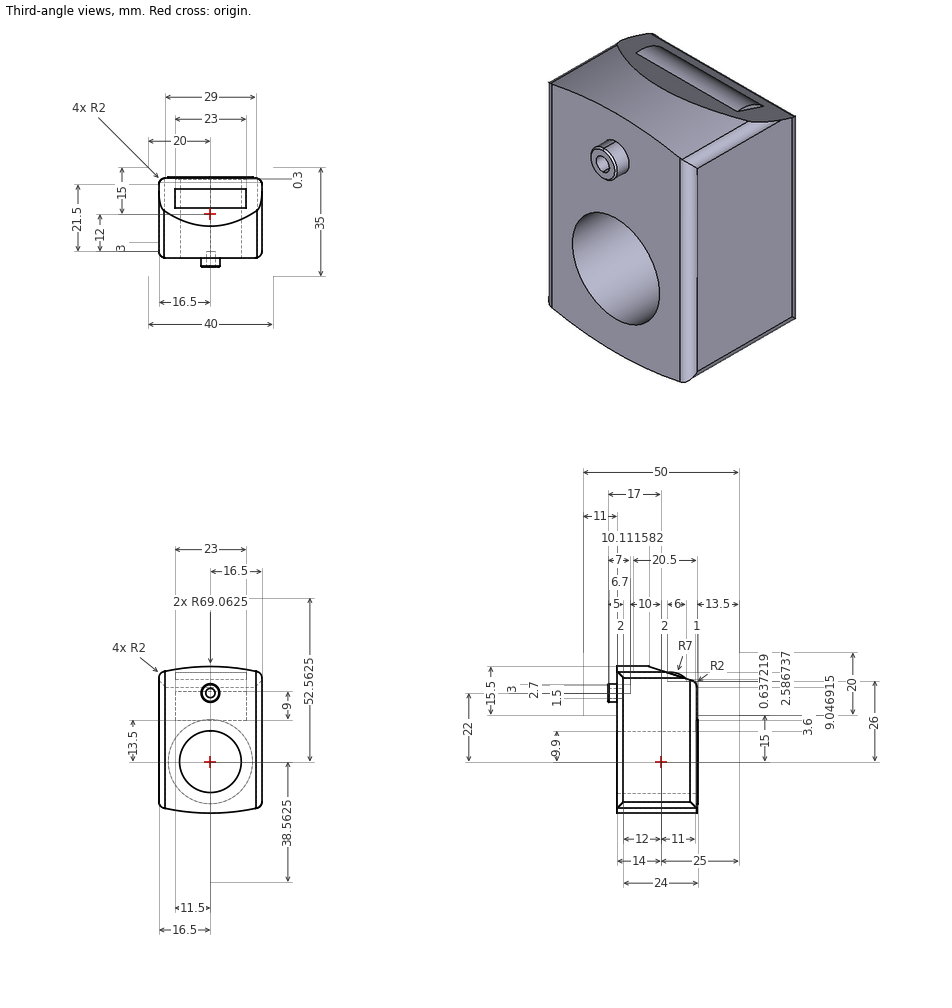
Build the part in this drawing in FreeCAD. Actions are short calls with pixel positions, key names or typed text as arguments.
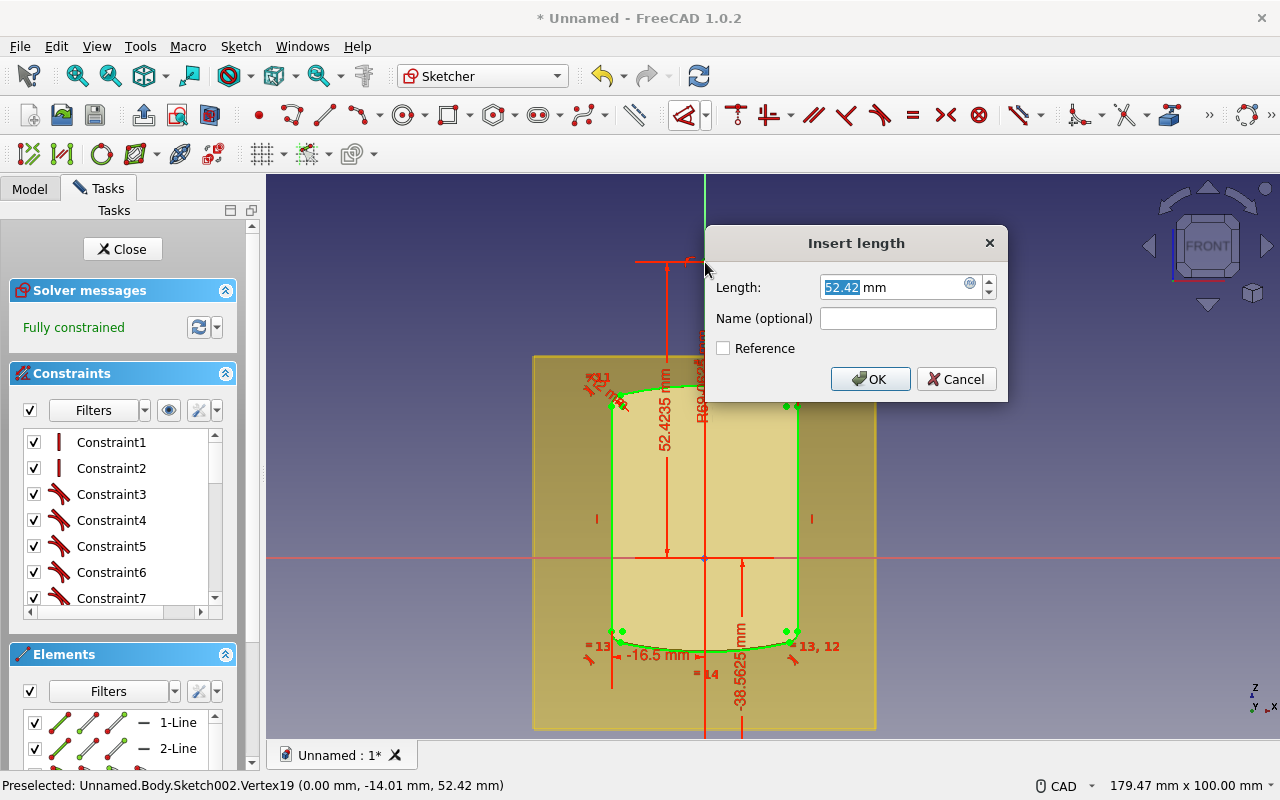
text(52.5625)
key(Return)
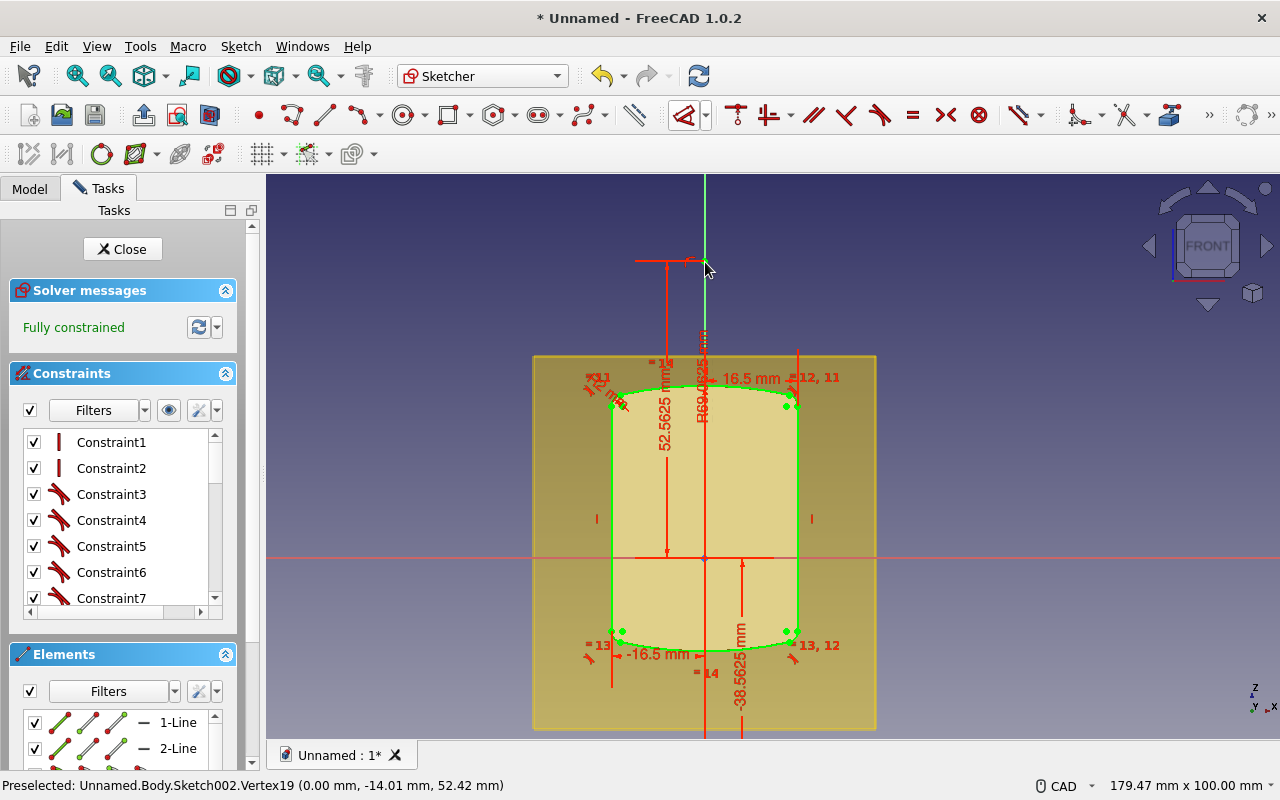
click(123, 249)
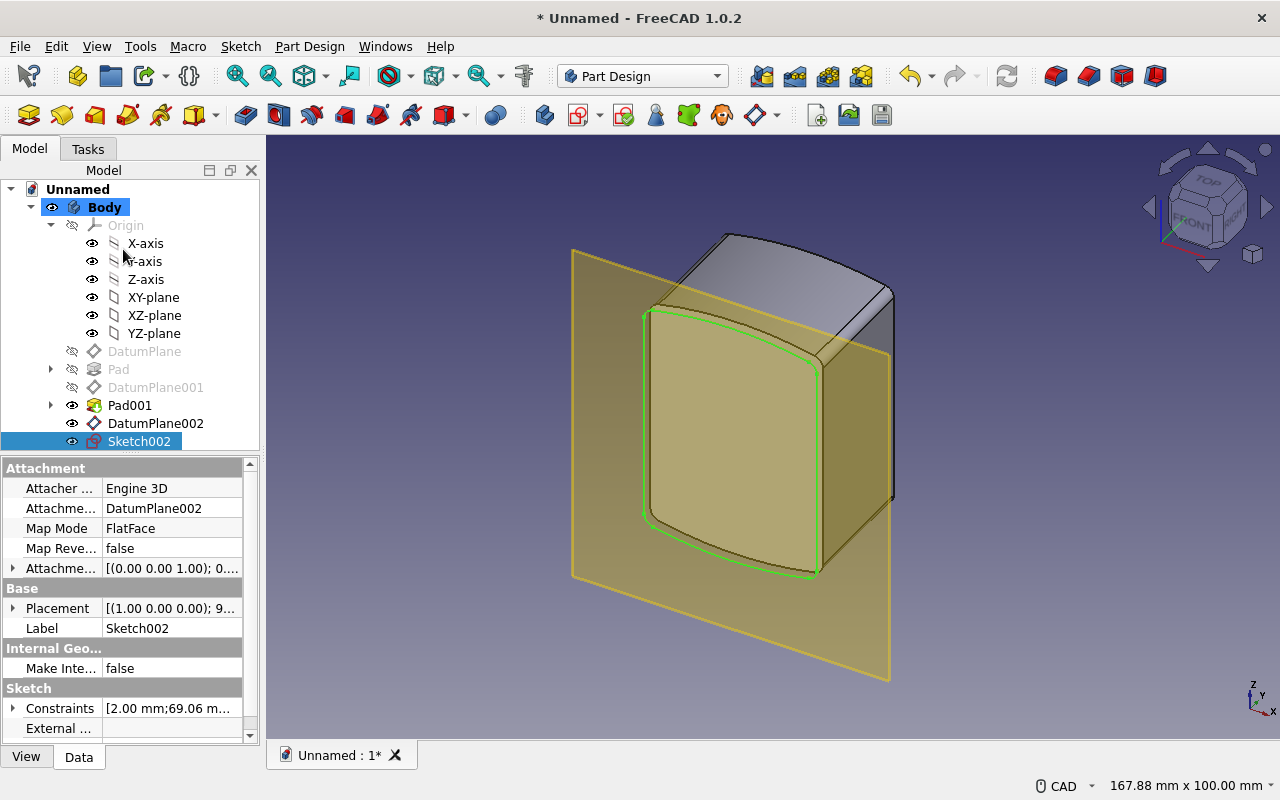
click(29, 116)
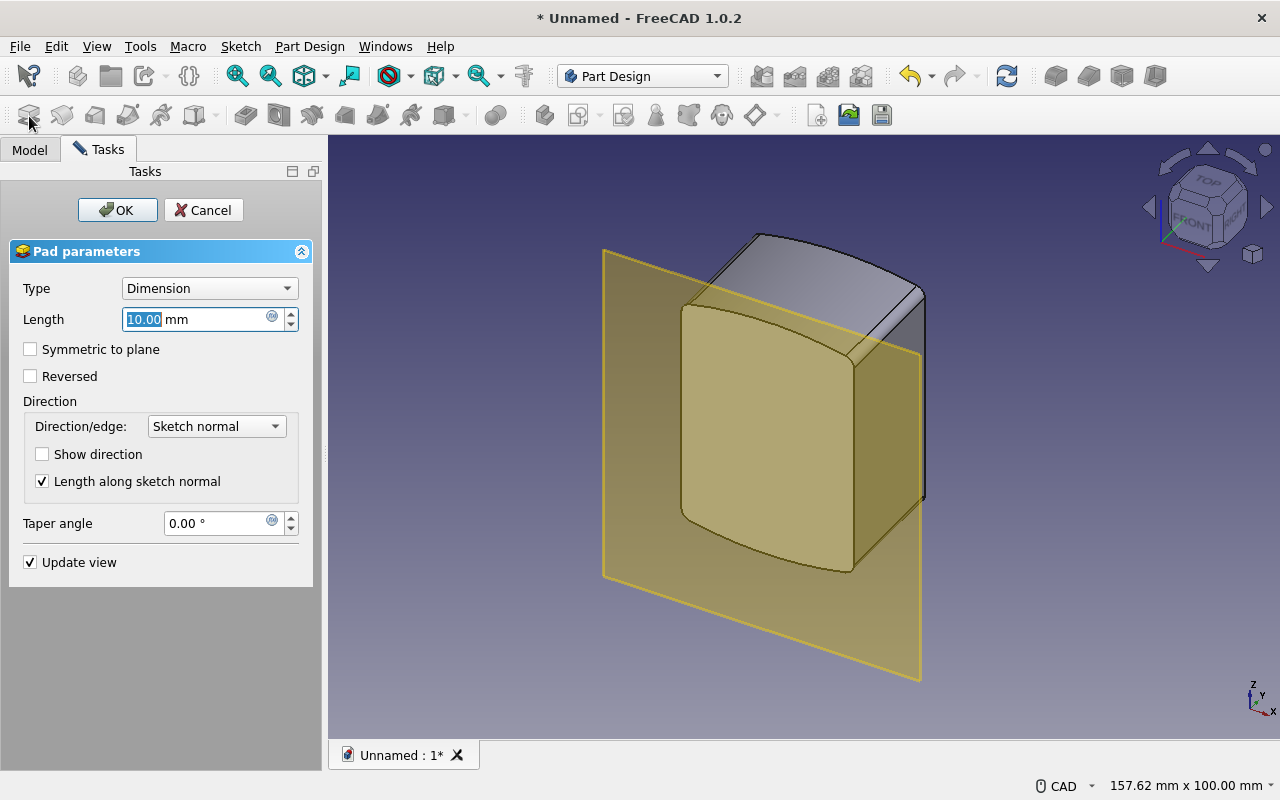
text(2)
key(Tab)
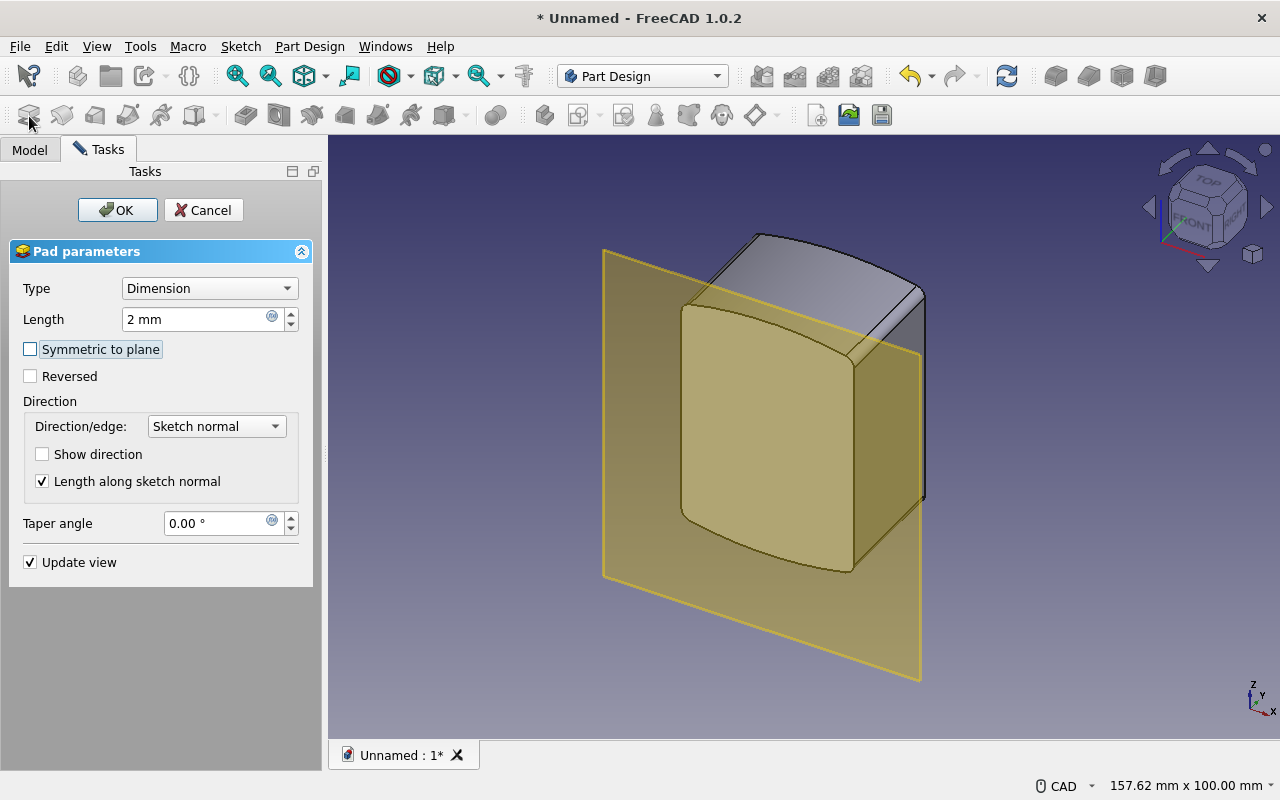
click(31, 376)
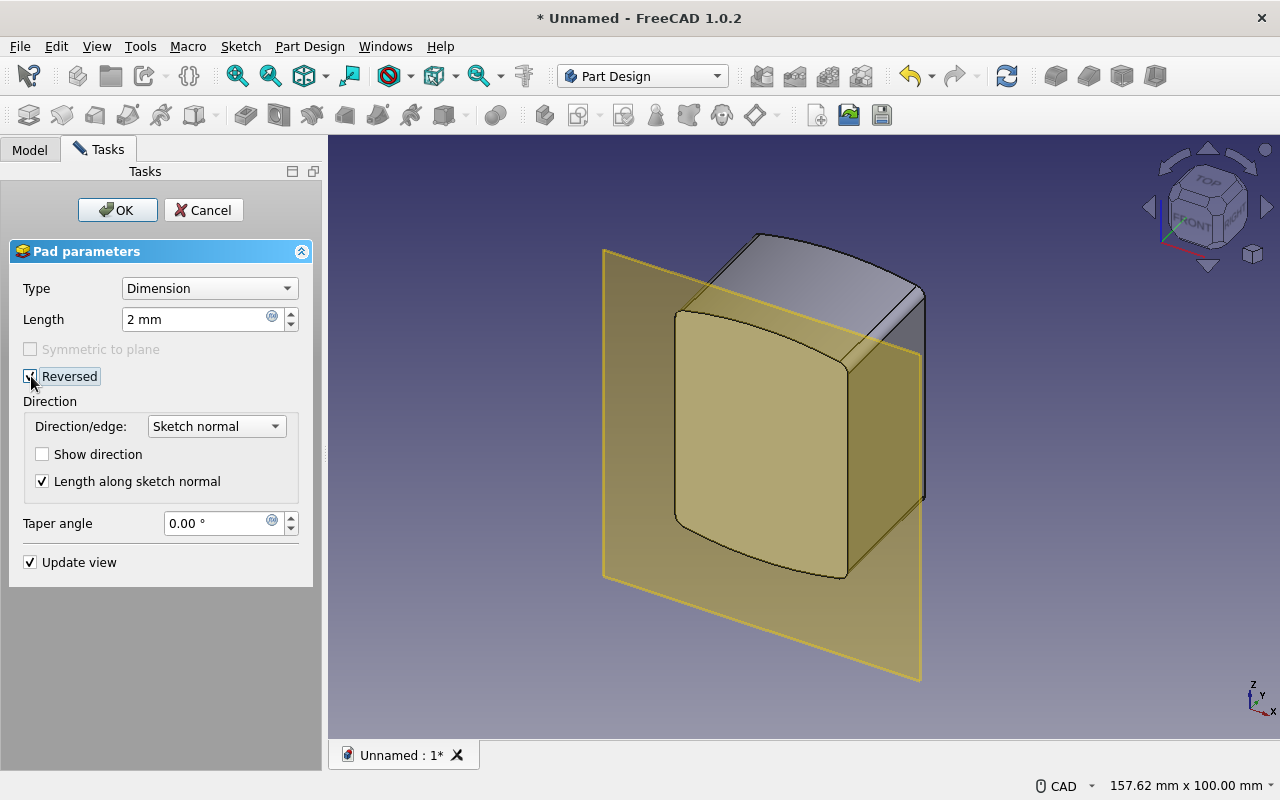
click(118, 210)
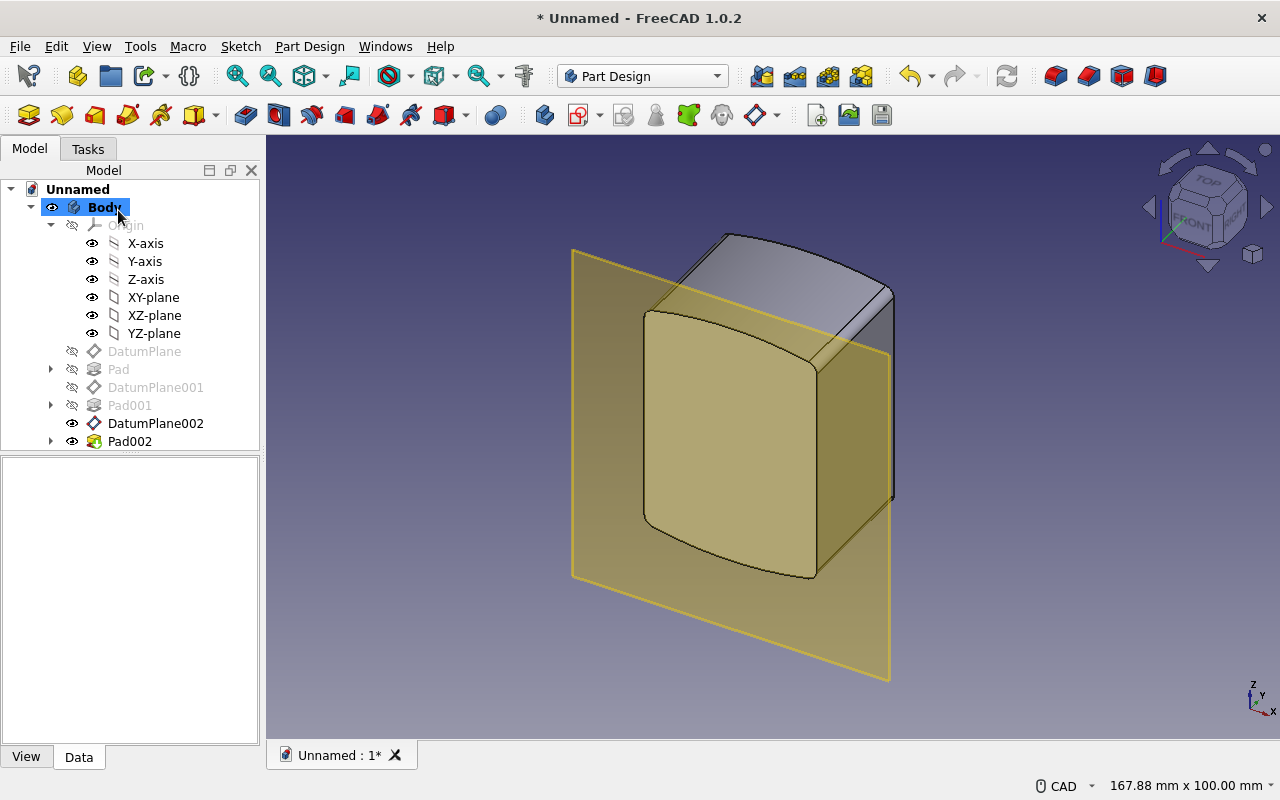
click(117, 423)
key(space)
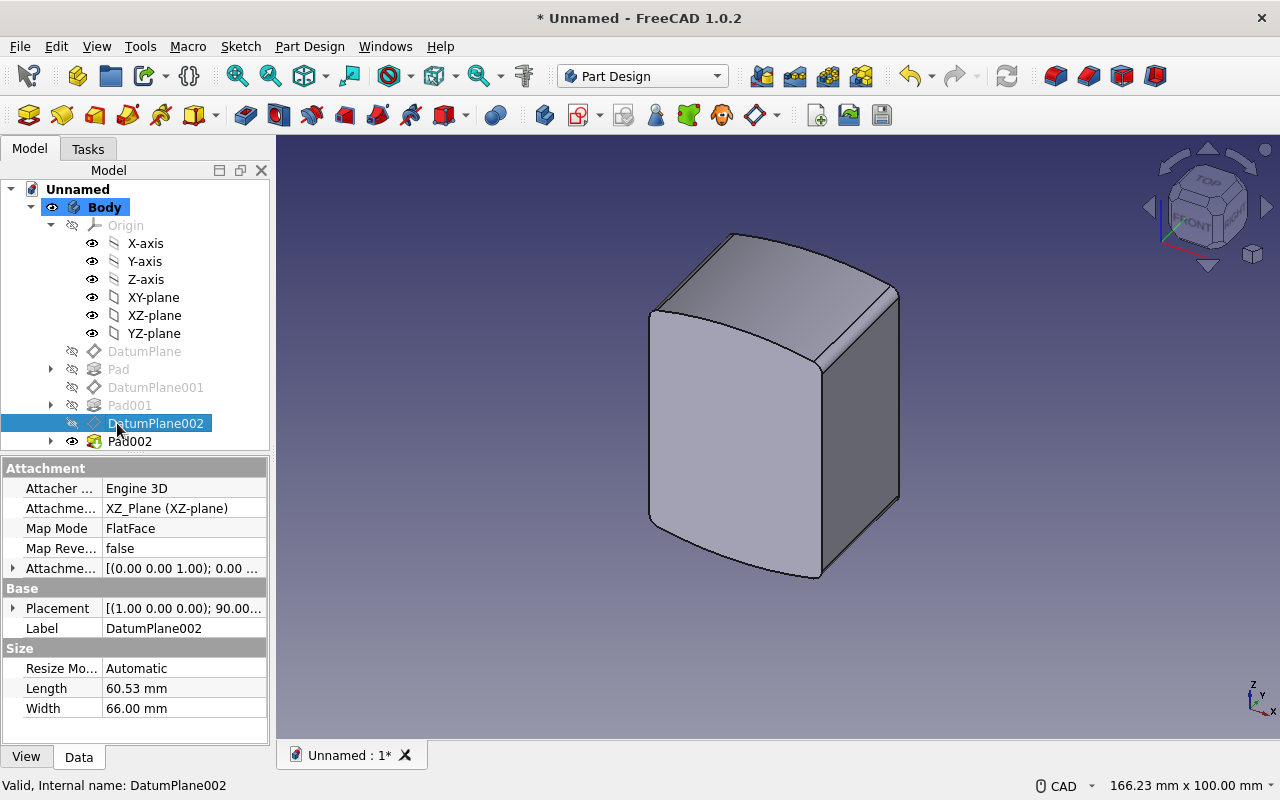
click(316, 699)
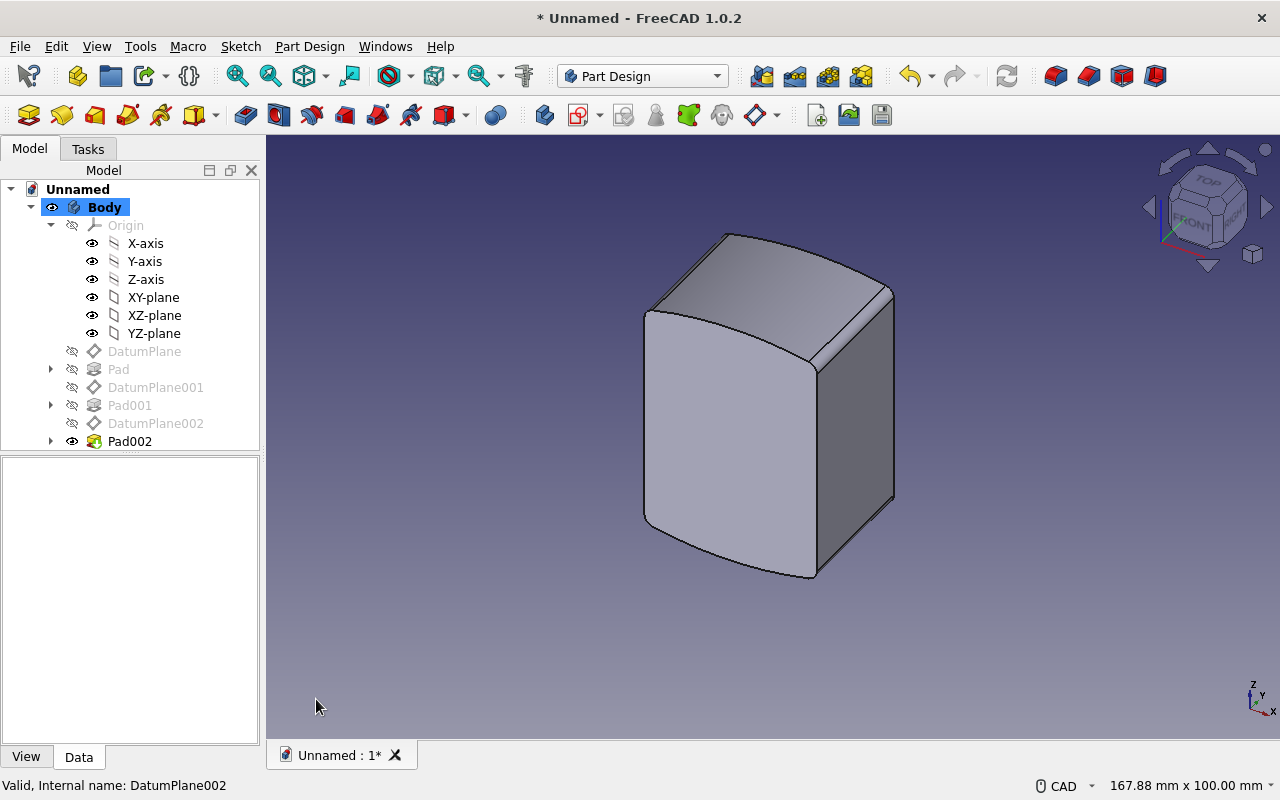
click(578, 116)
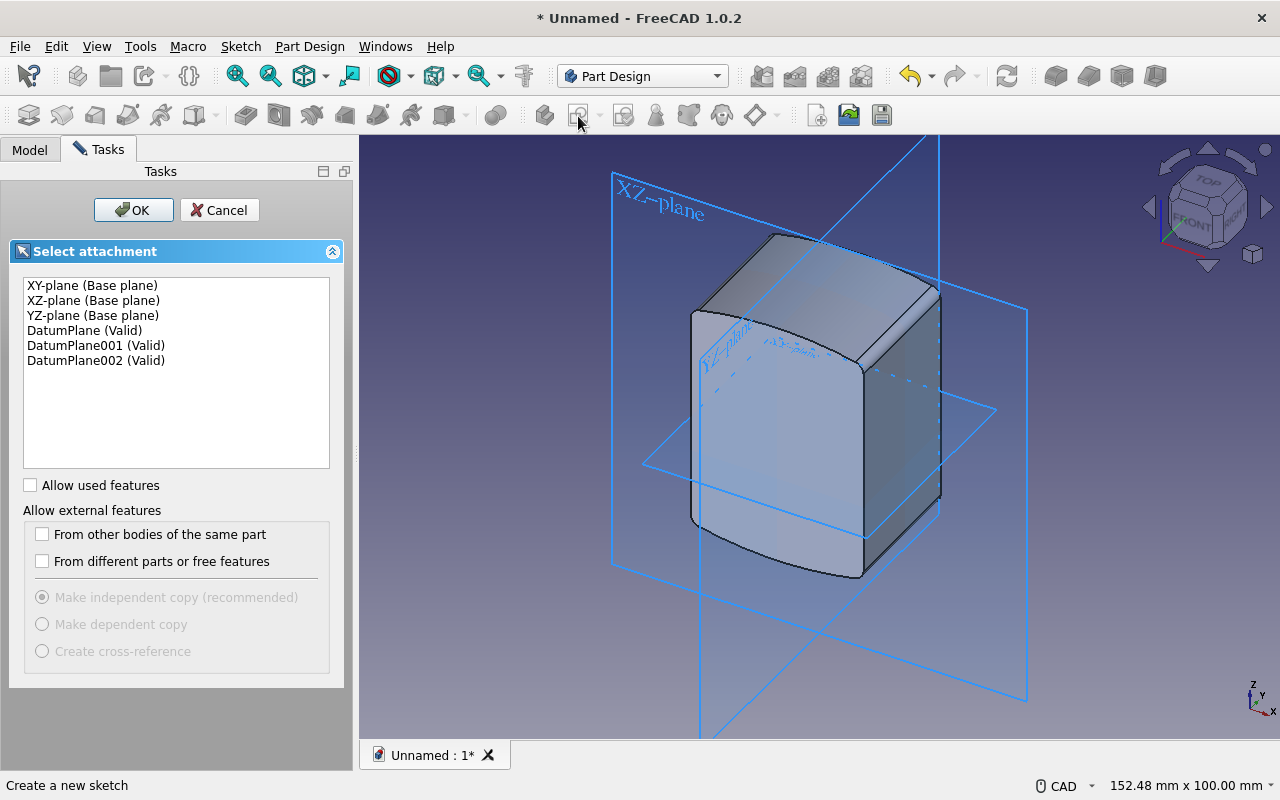
click(84, 286)